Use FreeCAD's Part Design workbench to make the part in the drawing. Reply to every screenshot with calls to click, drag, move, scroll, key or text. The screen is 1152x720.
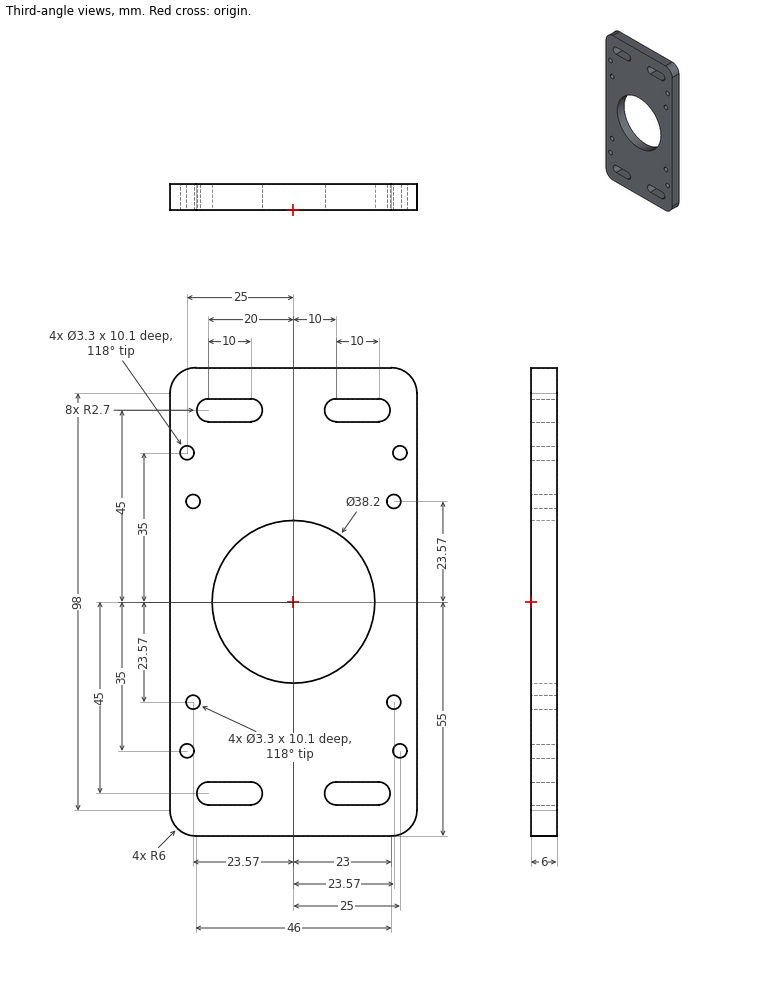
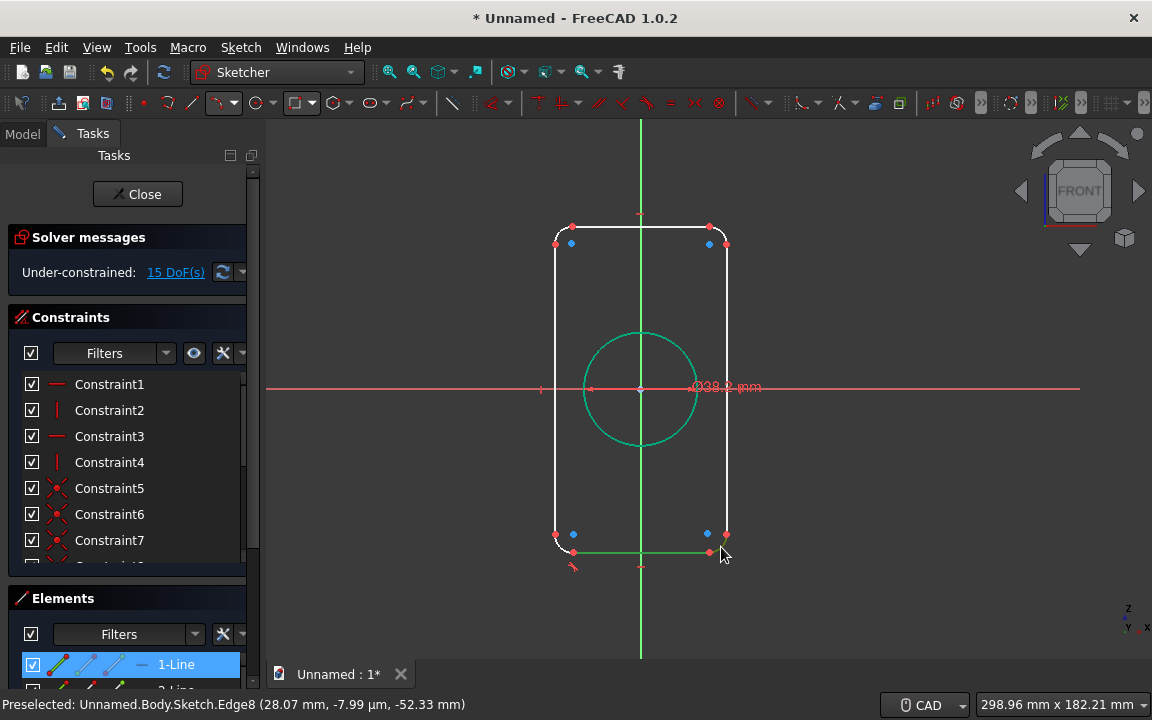
click(648, 104)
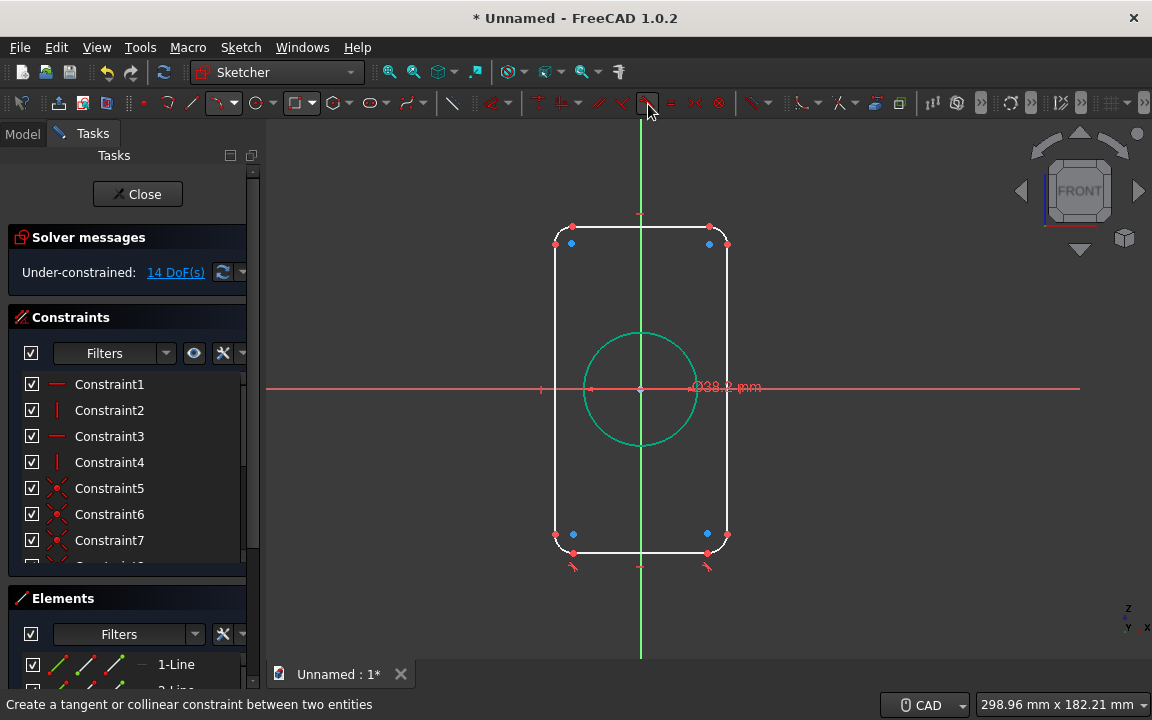
click(555, 448)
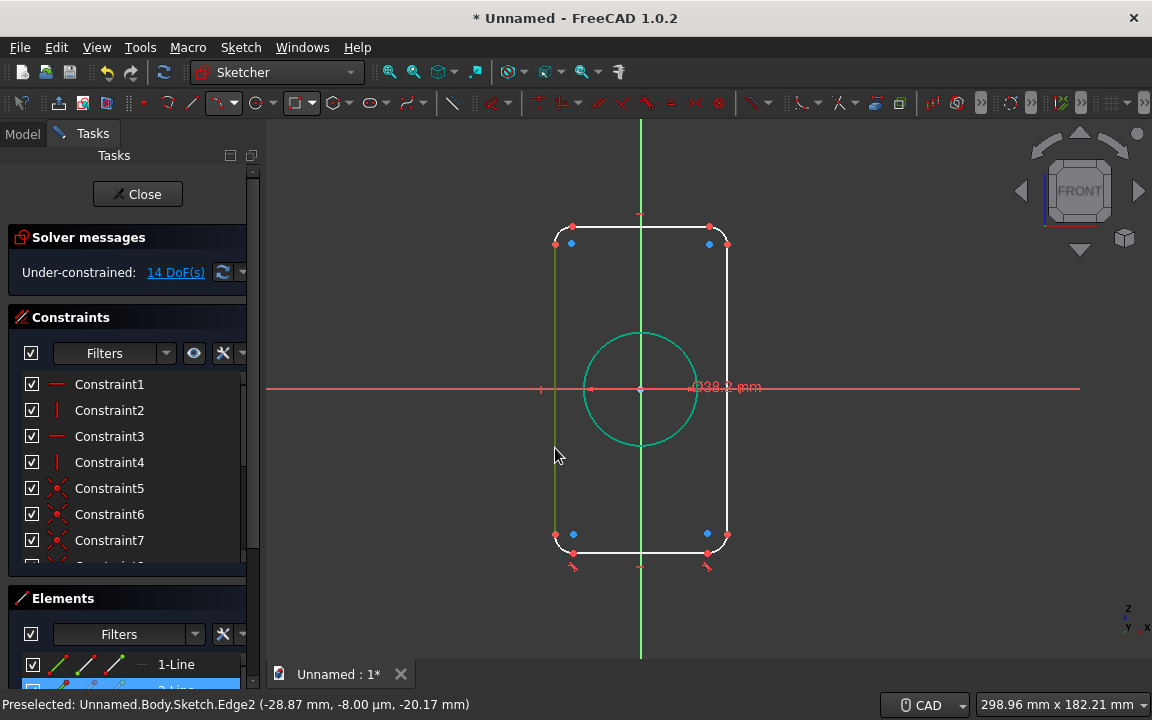
click(560, 548)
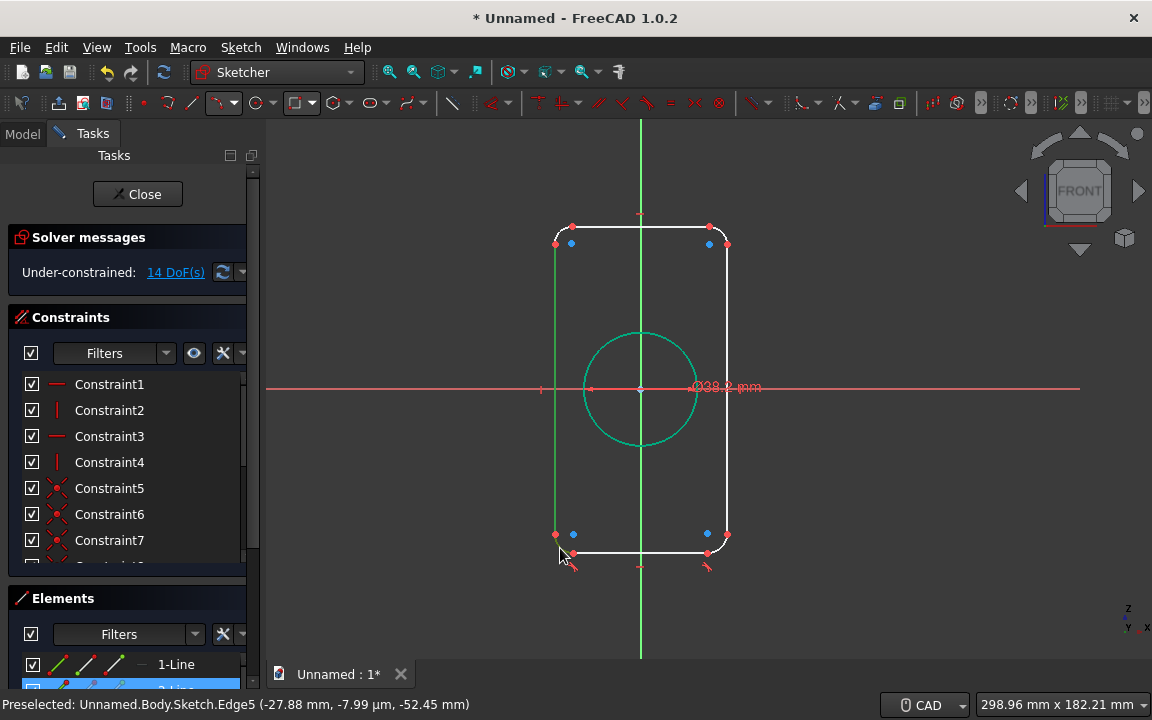
click(648, 104)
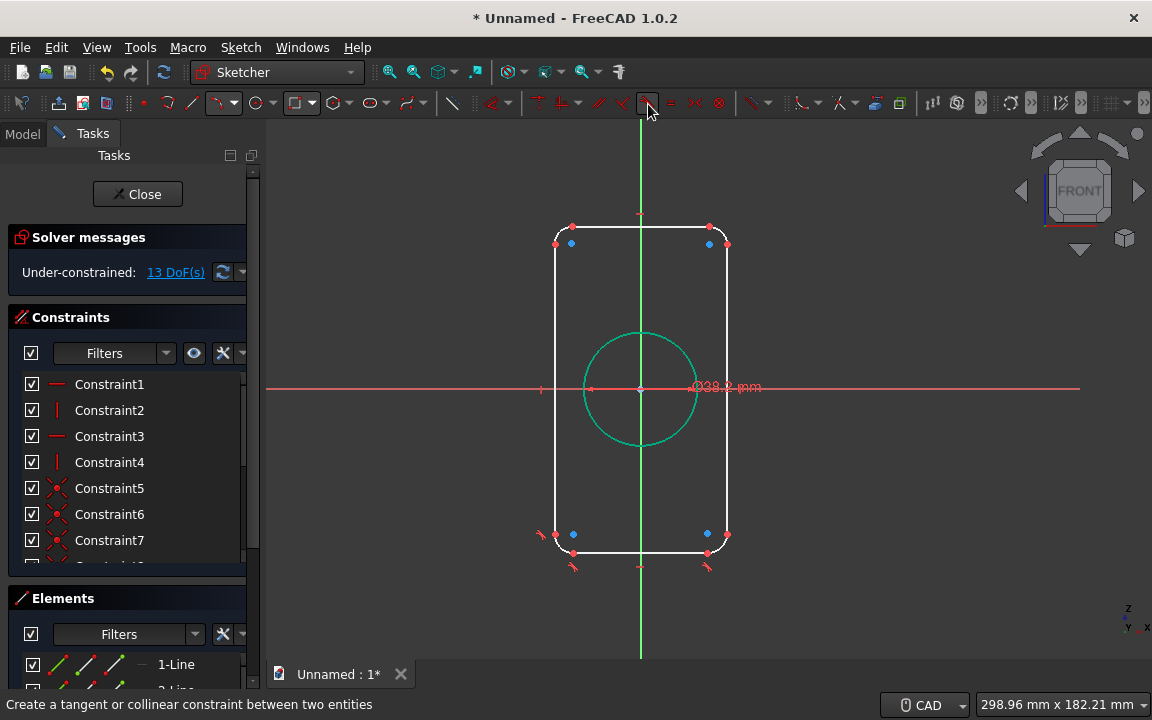
click(555, 448)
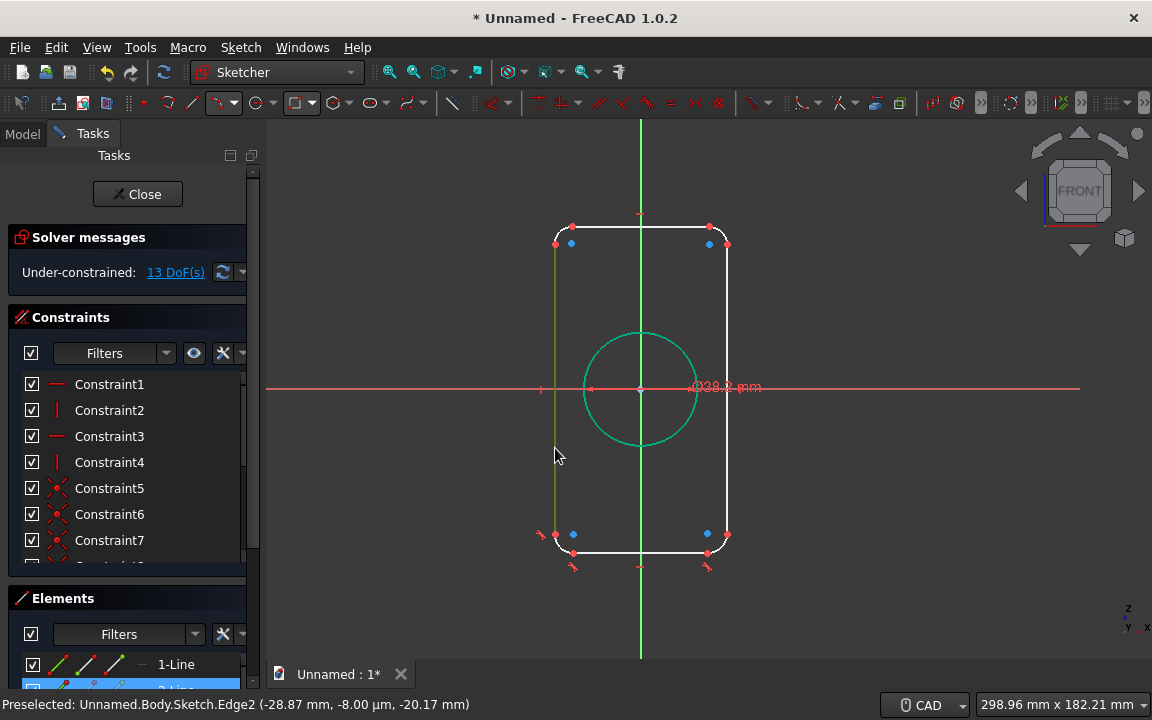
click(559, 232)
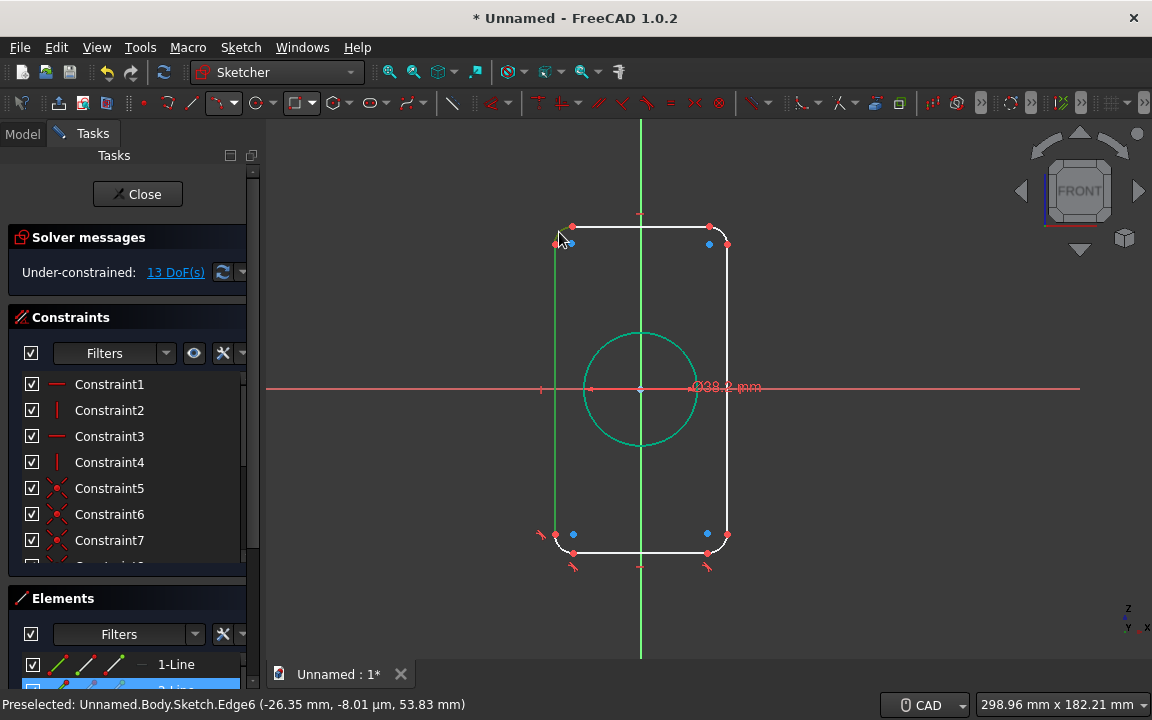
key(t)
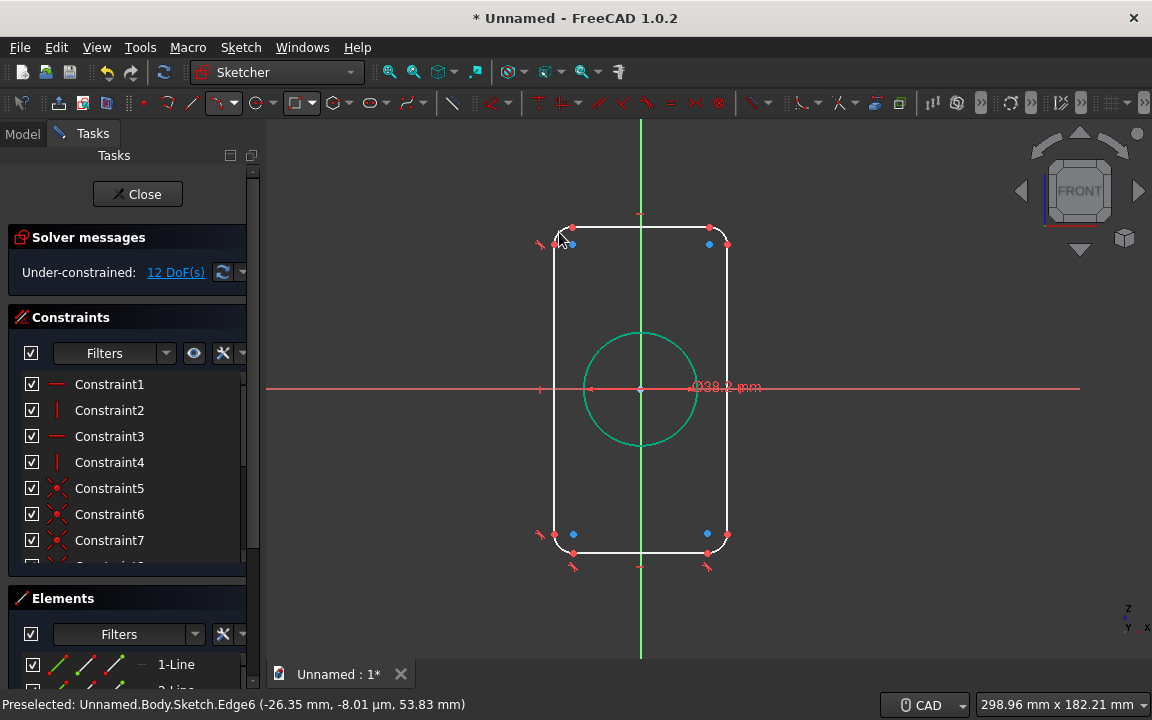
click(613, 227)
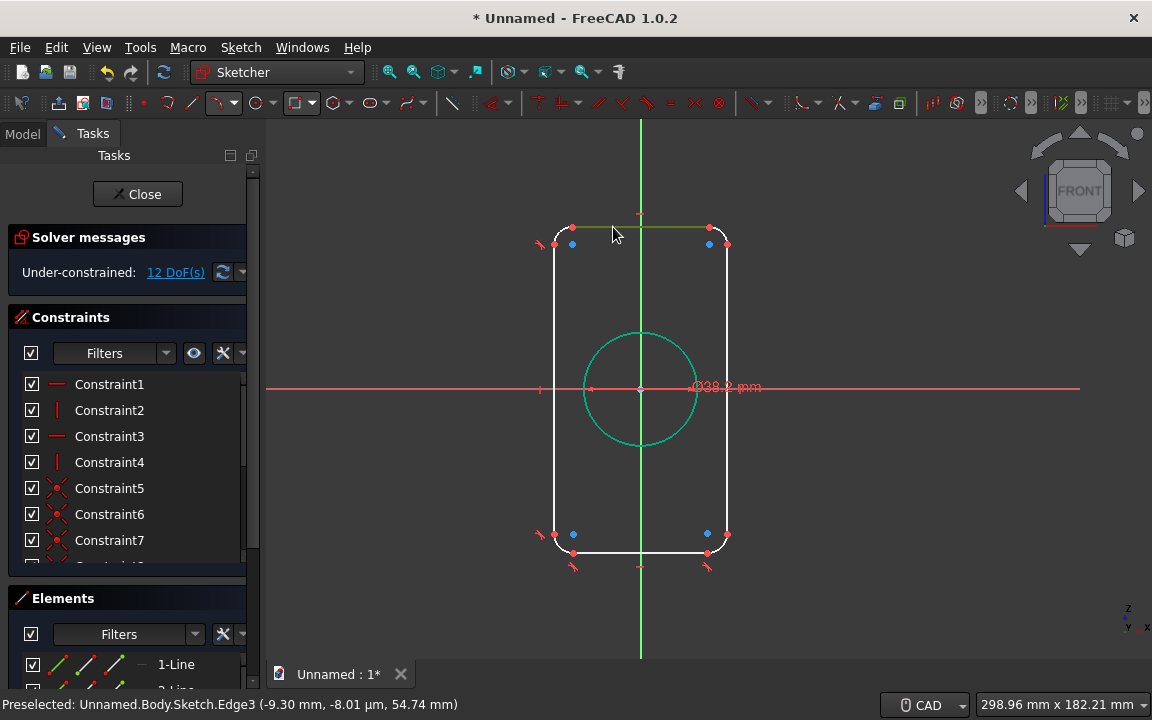
click(559, 232)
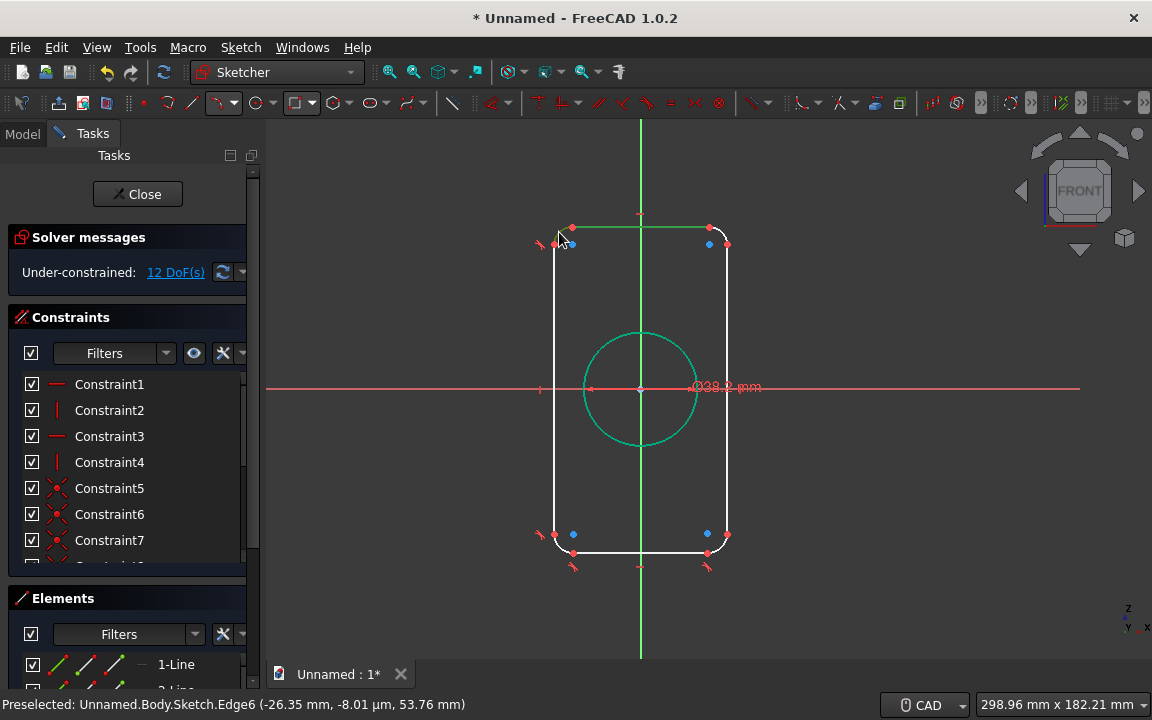
key(t)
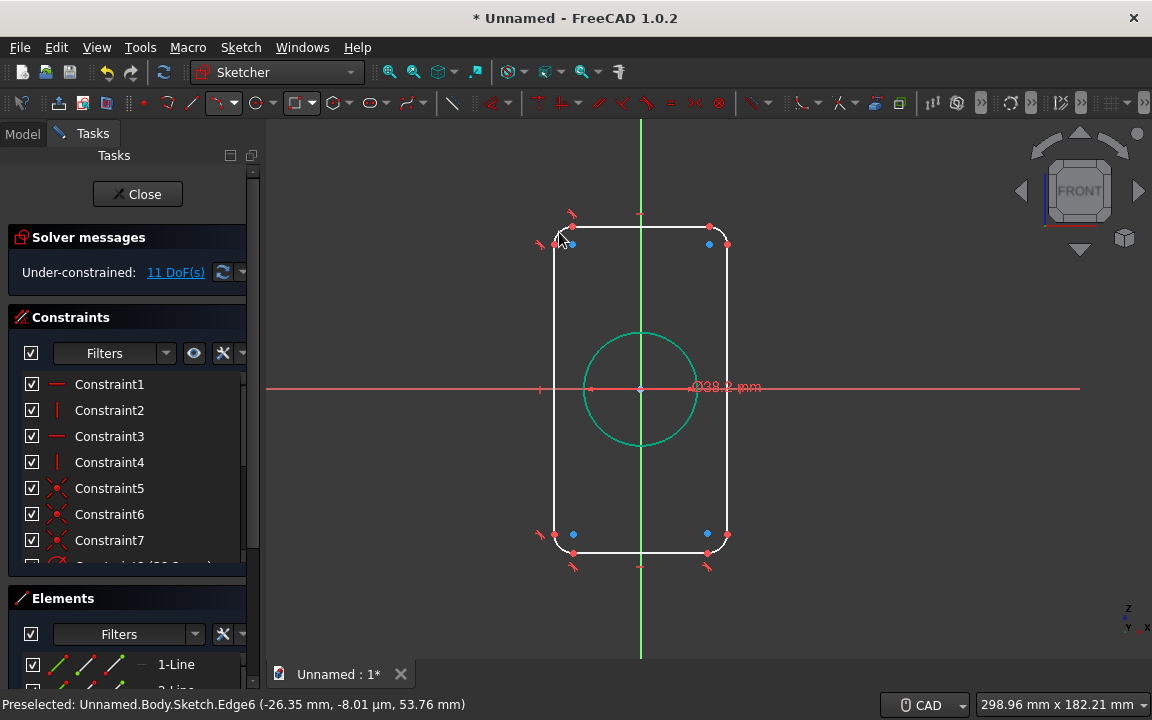
click(613, 227)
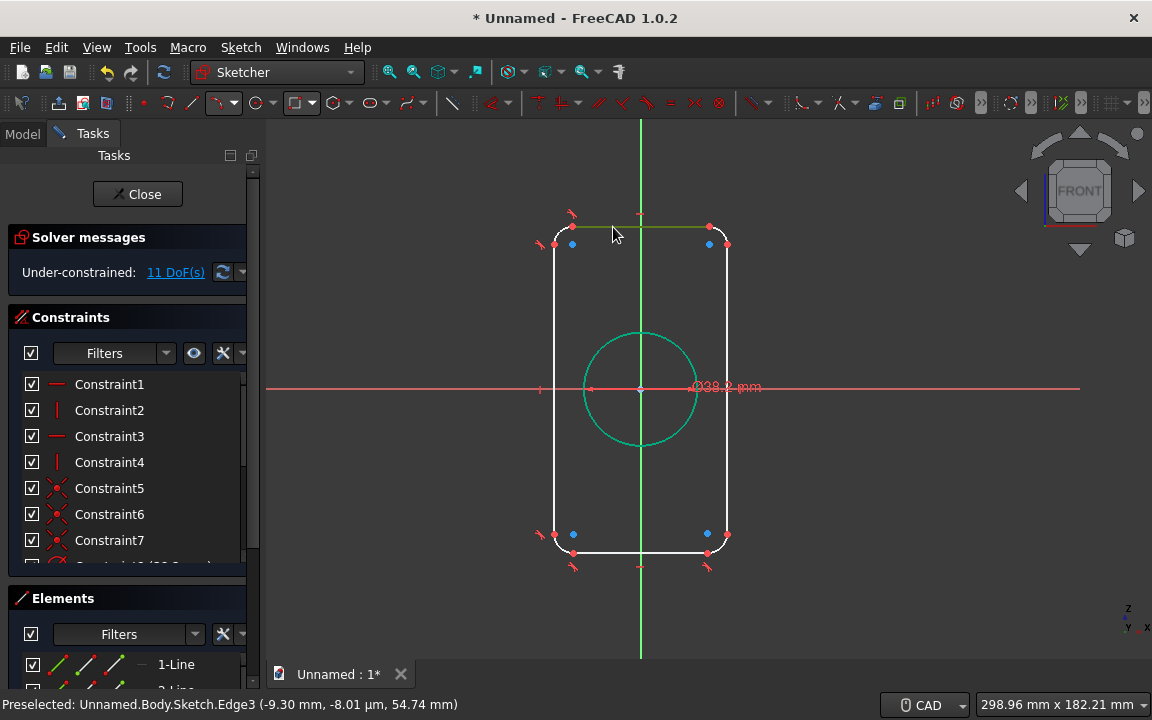
click(722, 232)